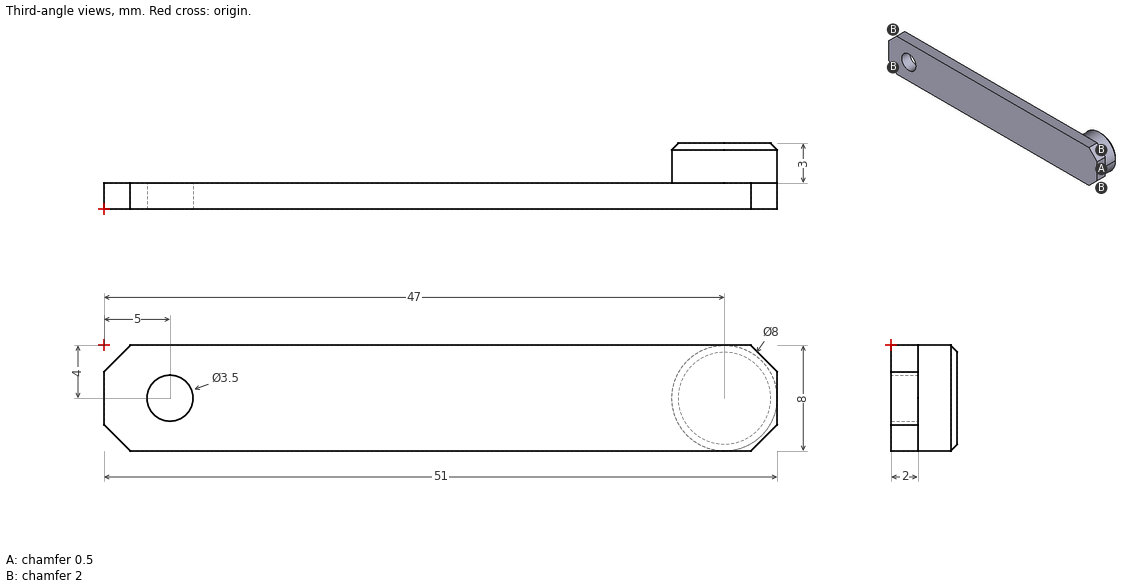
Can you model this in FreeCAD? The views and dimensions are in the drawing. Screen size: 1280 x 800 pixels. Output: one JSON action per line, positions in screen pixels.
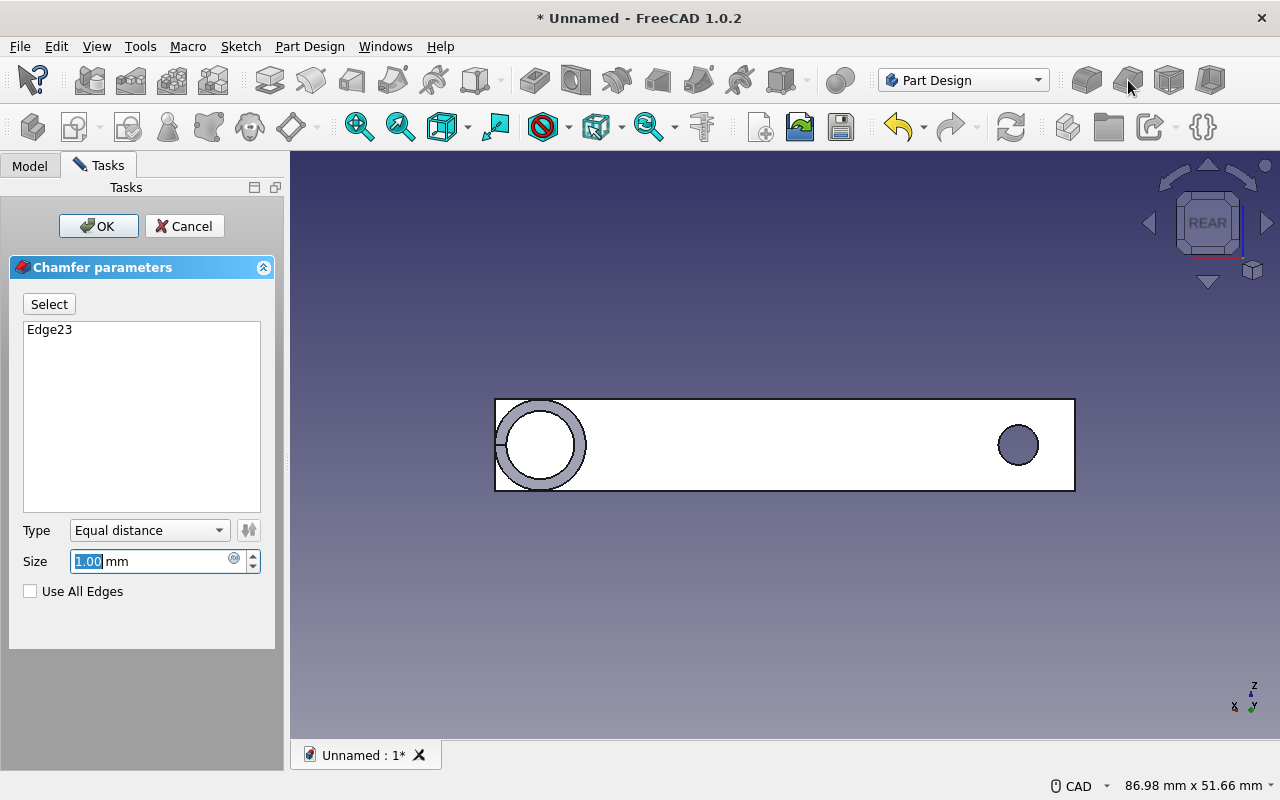
{"action": "type", "text": "0.5"}
{"action": "key", "text": "Tab"}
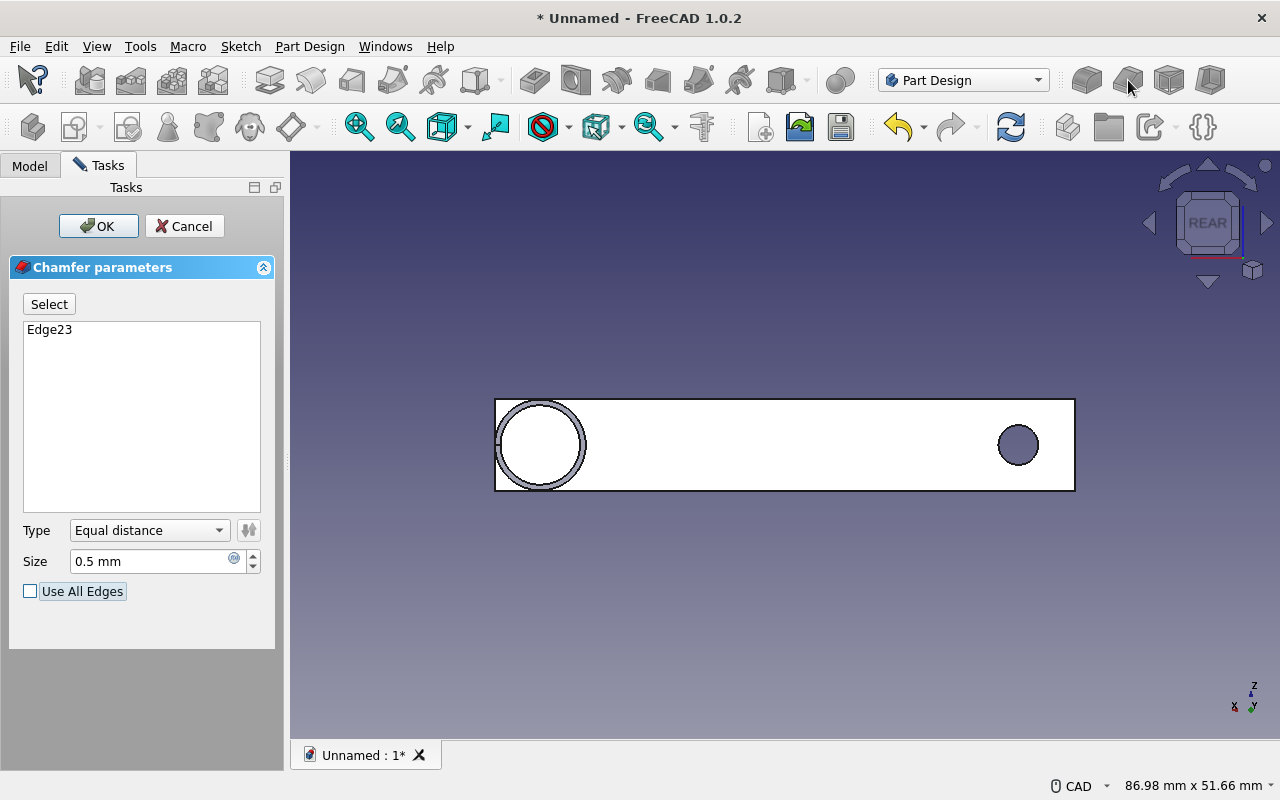
{"action": "left_click", "coordinate": [99, 226]}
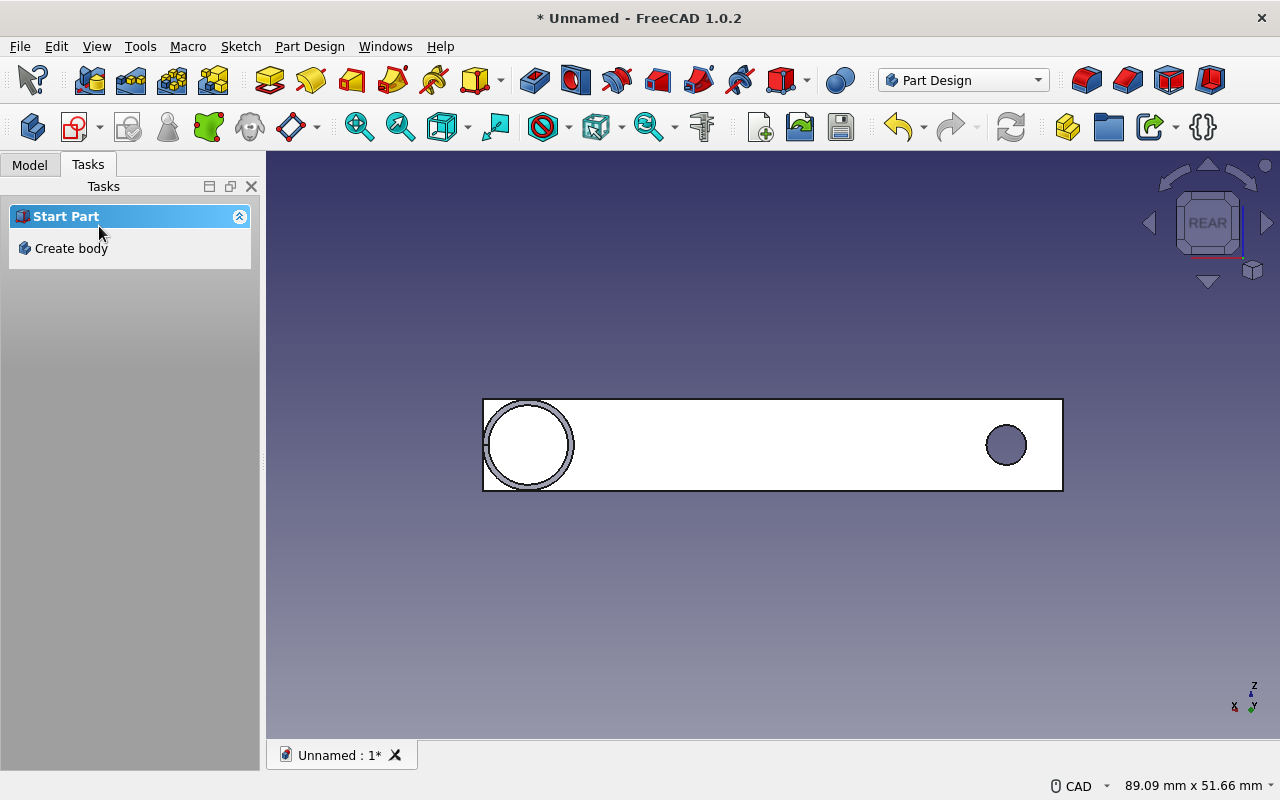
{"action": "key", "text": "0"}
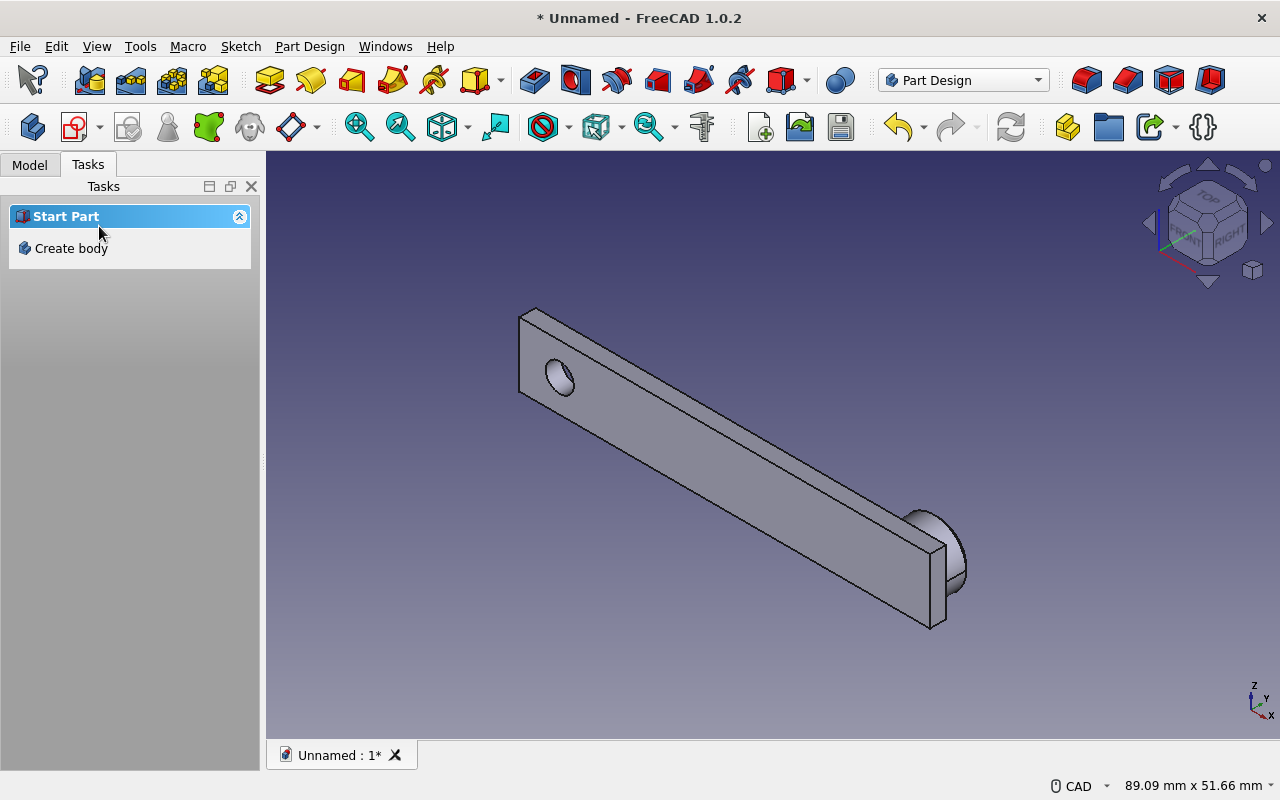
{"action": "left_click", "coordinate": [938, 549]}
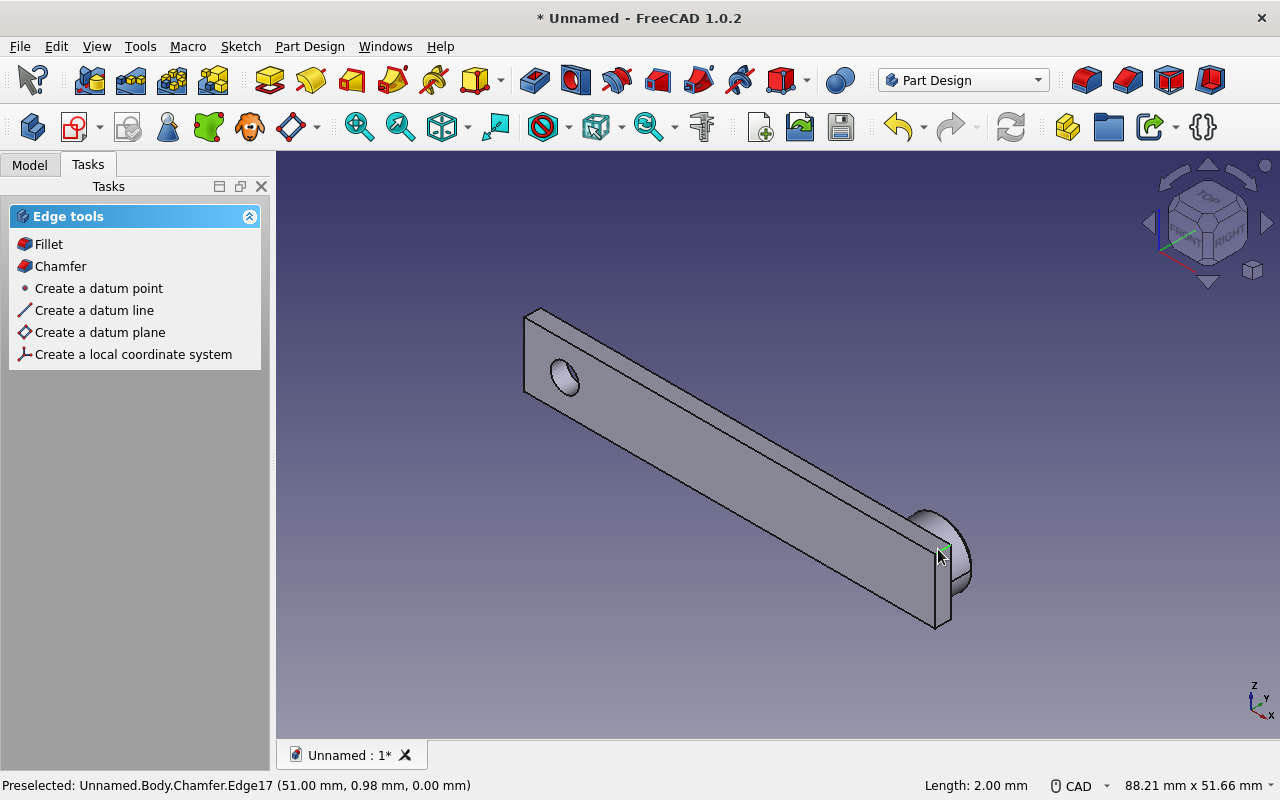
{"action": "key", "text": "2"}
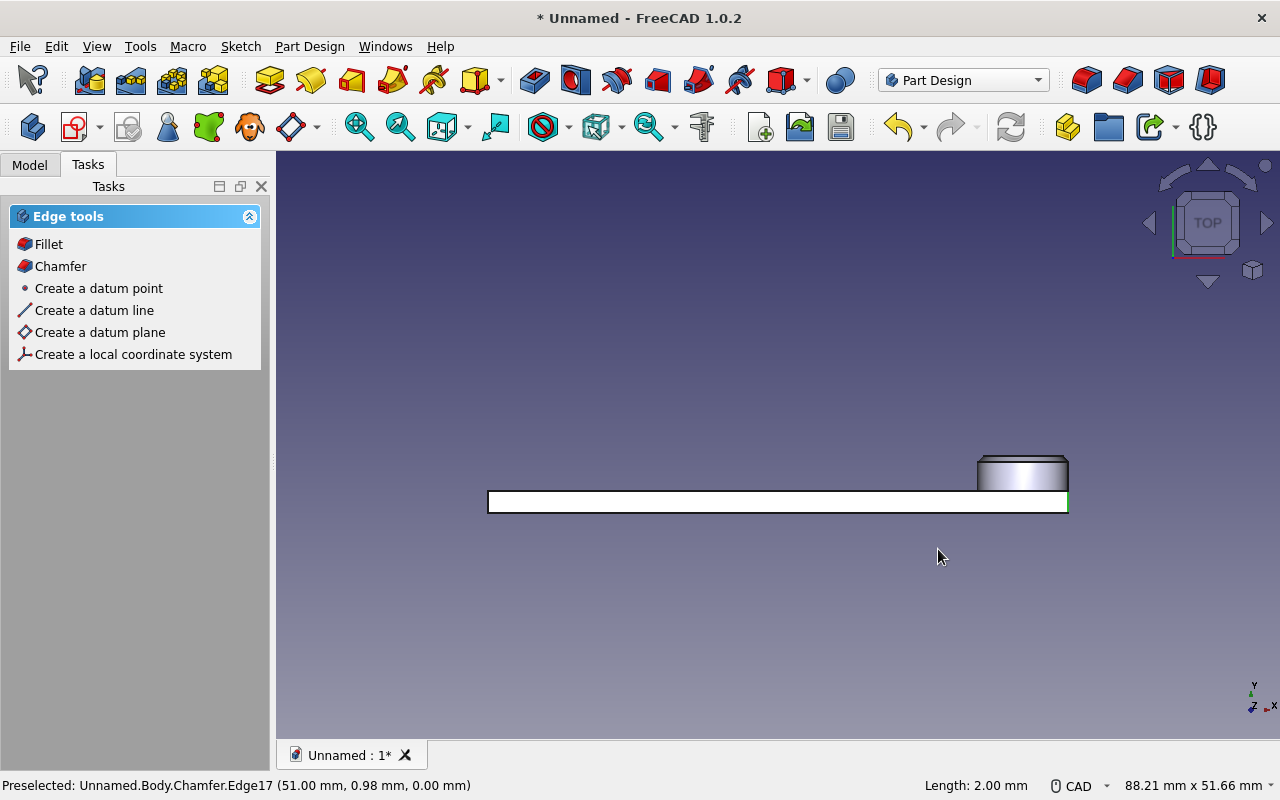
{"action": "left_click", "coordinate": [488, 499], "text": "ctrl"}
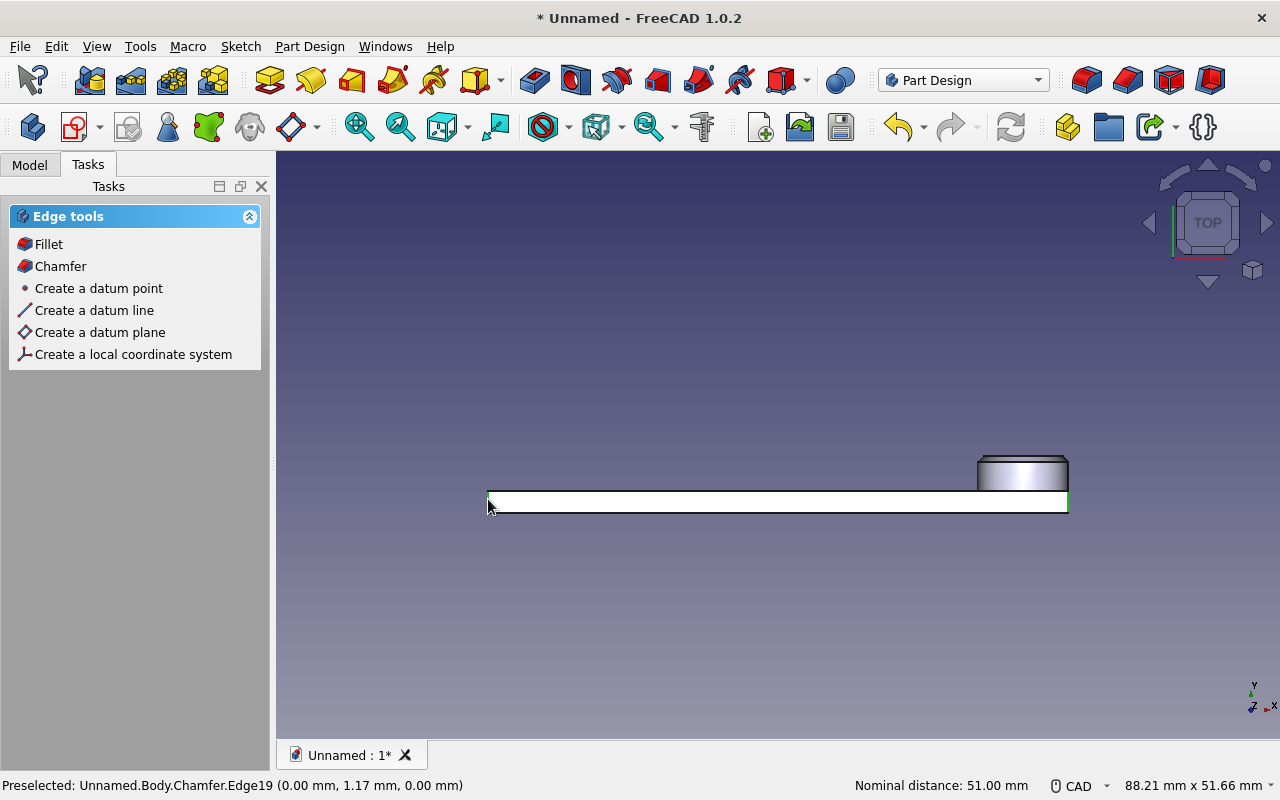
{"action": "key", "text": "1"}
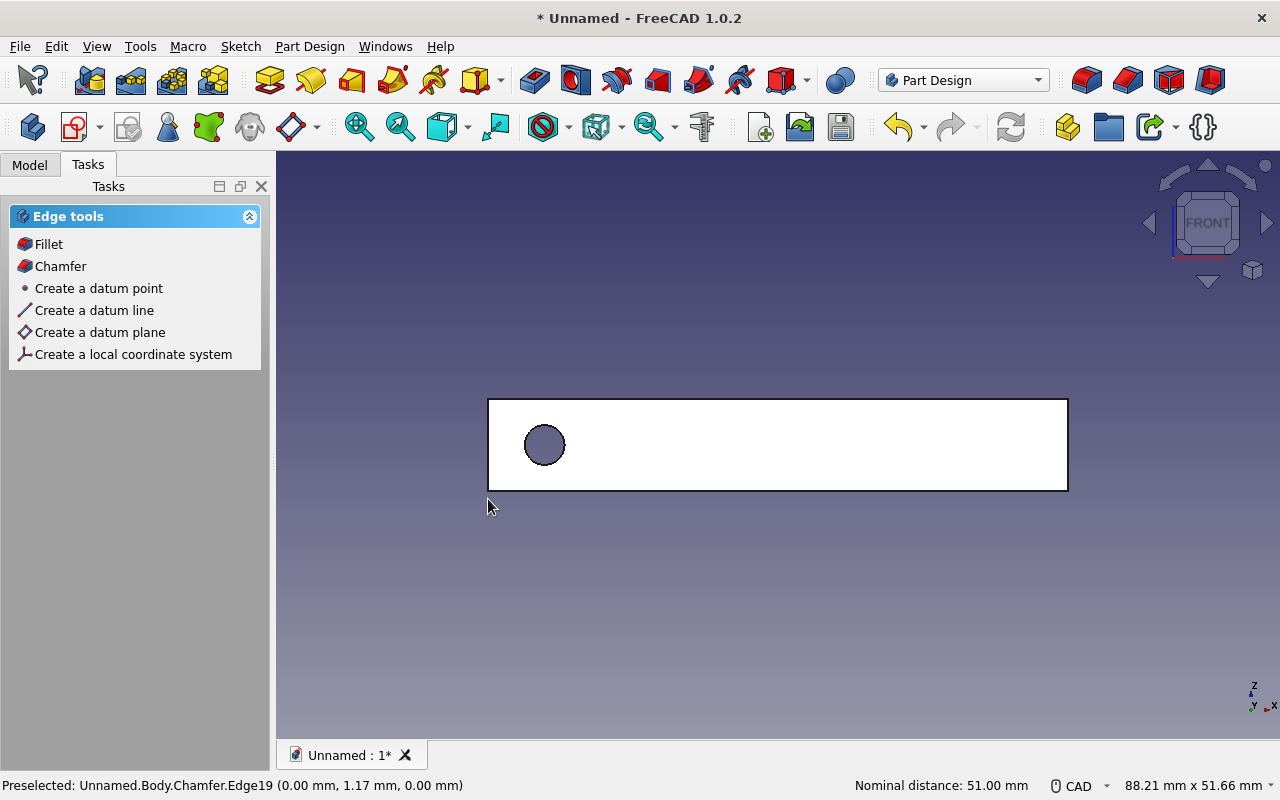
{"action": "key", "text": "3"}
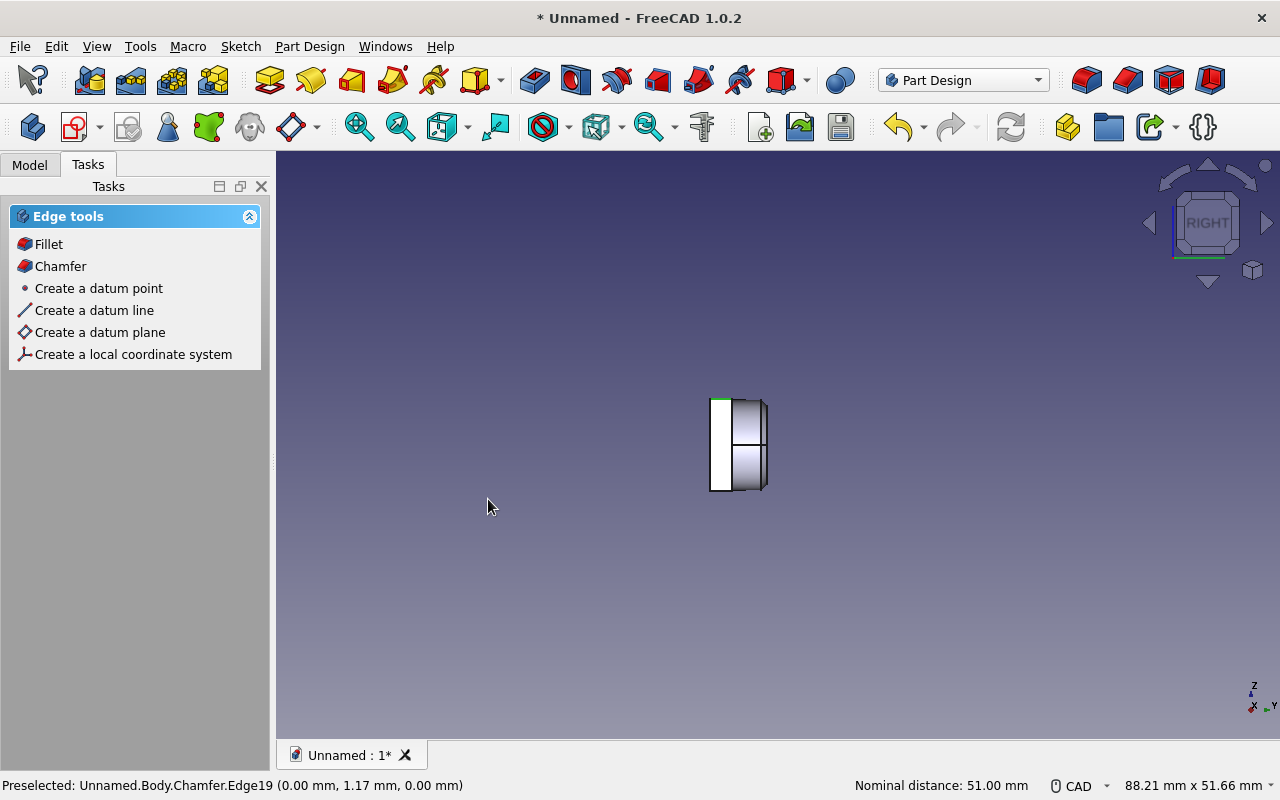
{"action": "key", "text": "v f"}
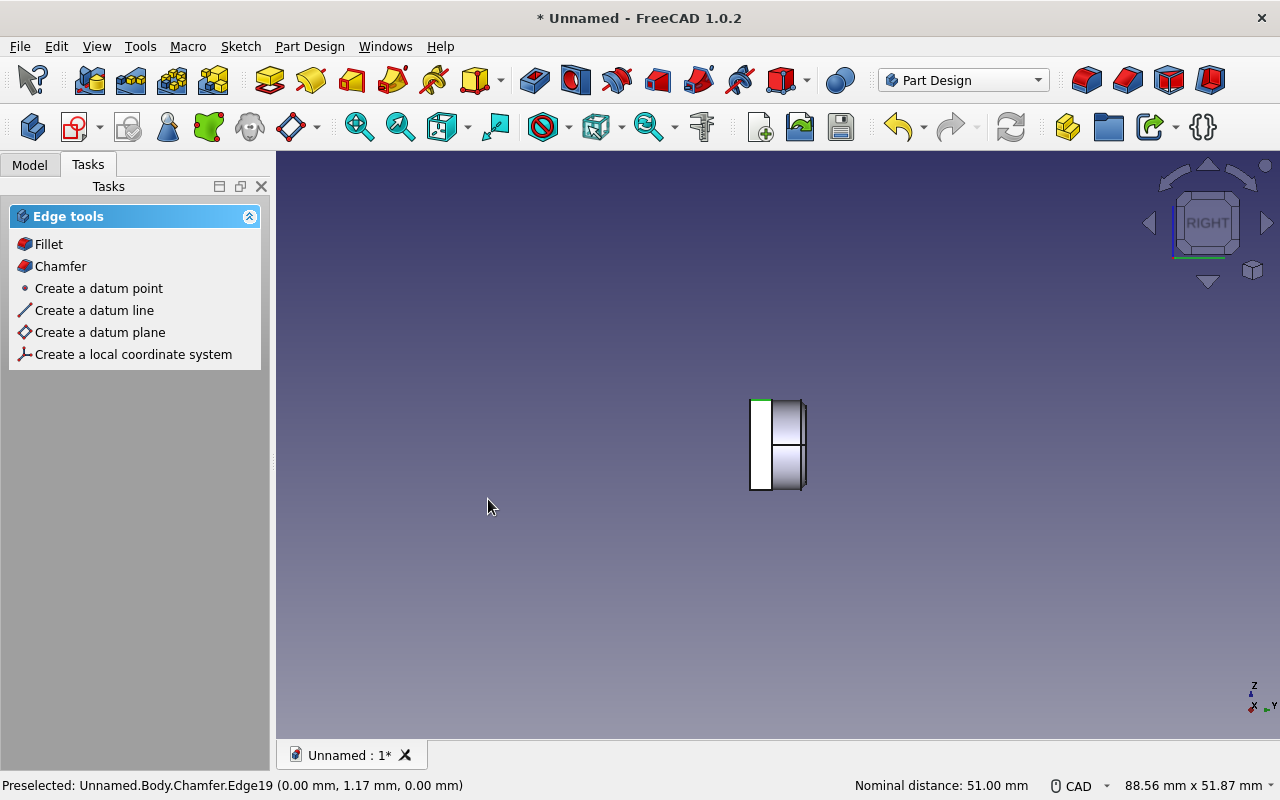
{"action": "left_click", "coordinate": [761, 489], "text": "ctrl"}